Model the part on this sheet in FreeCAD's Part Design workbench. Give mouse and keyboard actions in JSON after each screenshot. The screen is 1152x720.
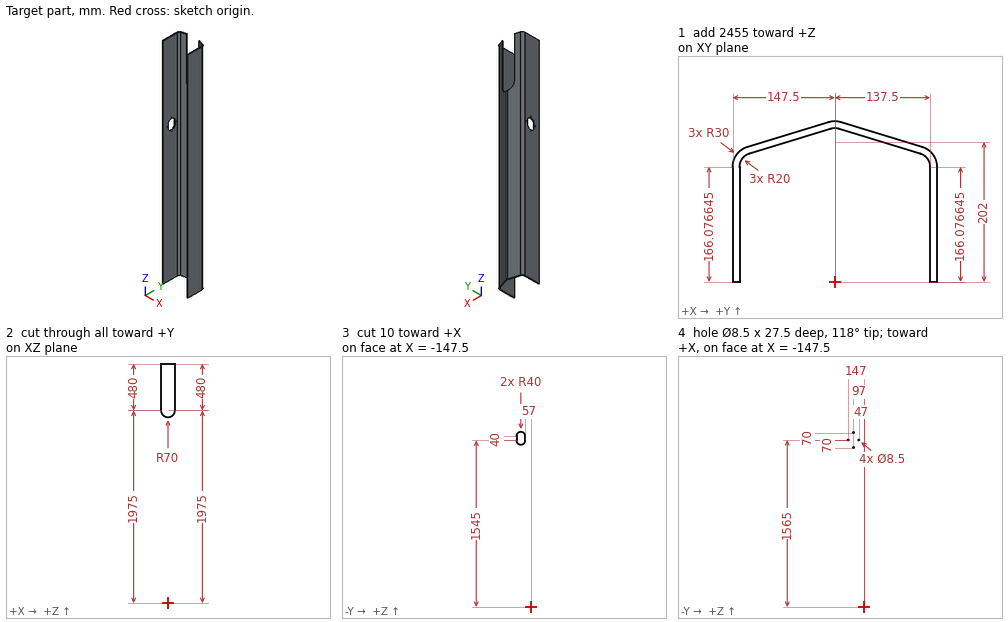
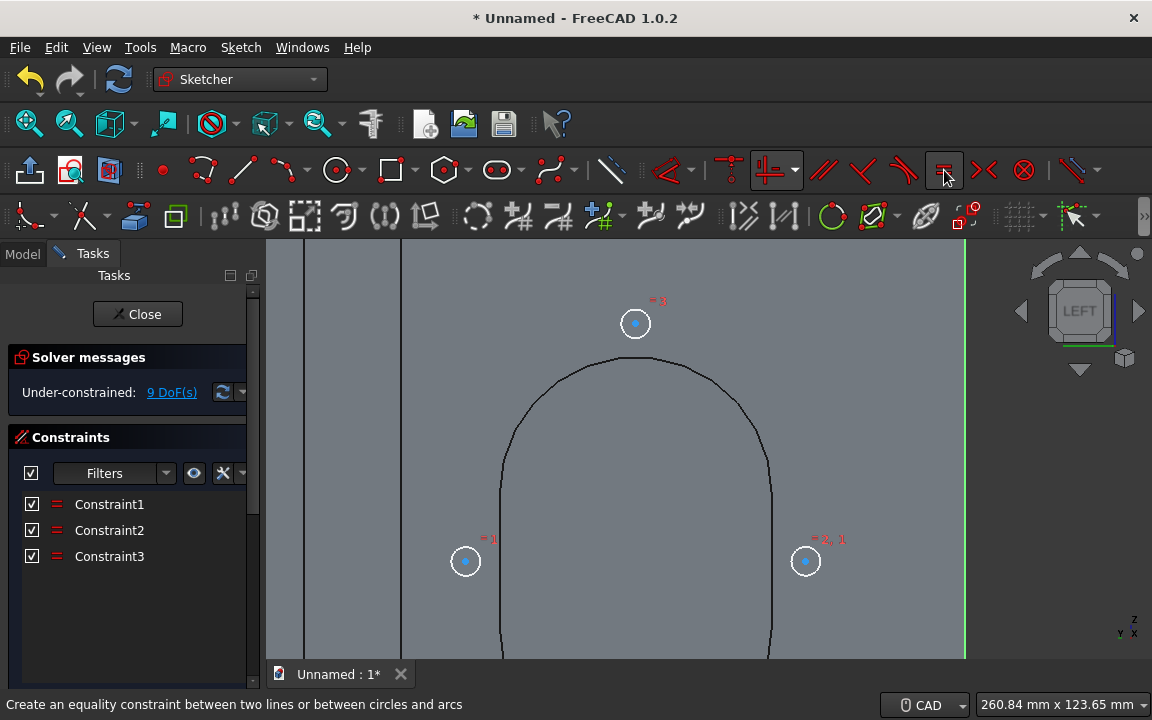
{"action": "left_click", "coordinate": [466, 561]}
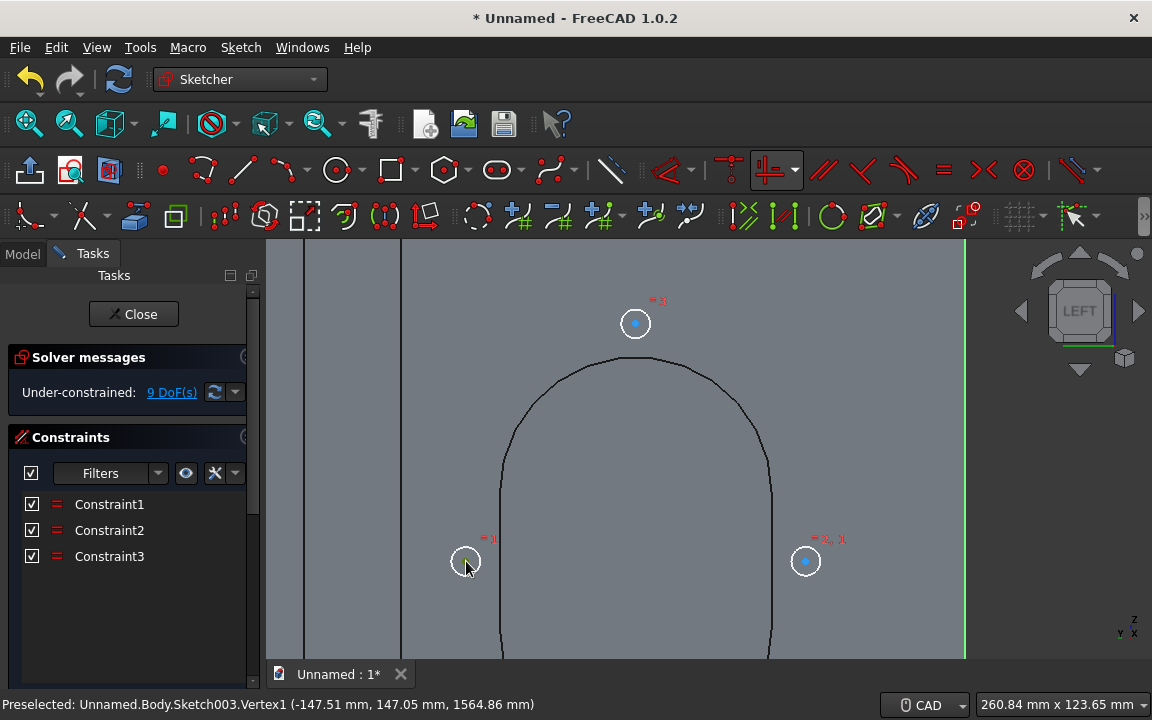
{"action": "left_click", "coordinate": [806, 561]}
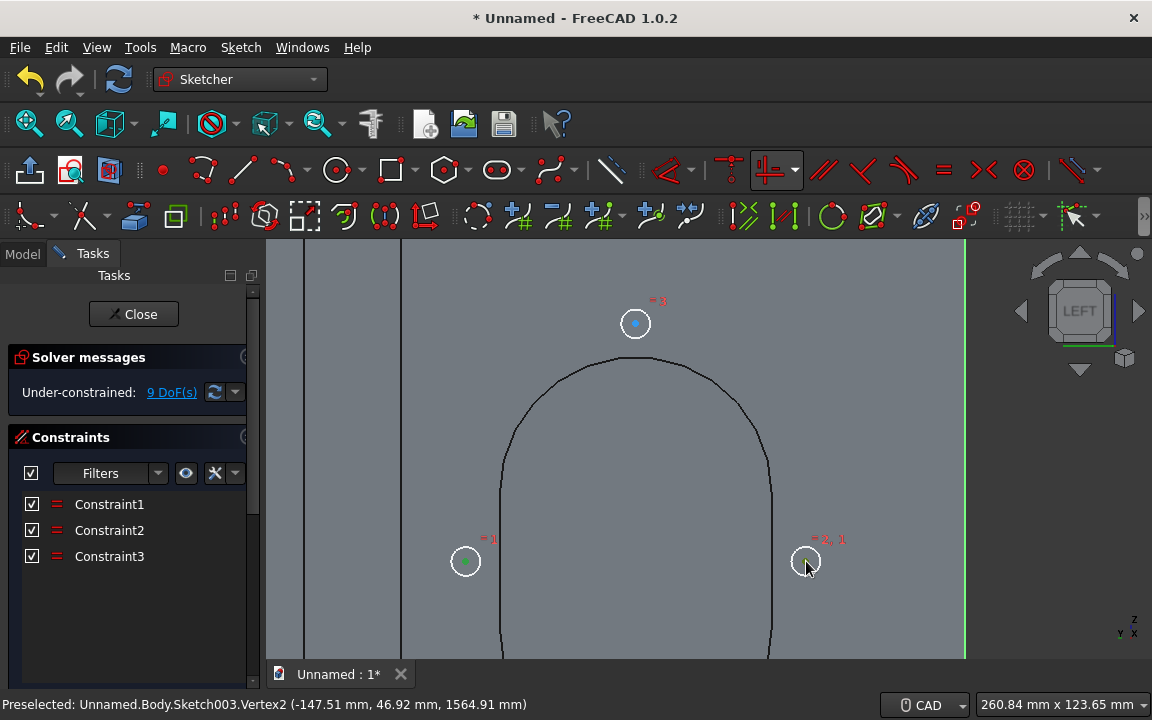
{"action": "key", "text": "h"}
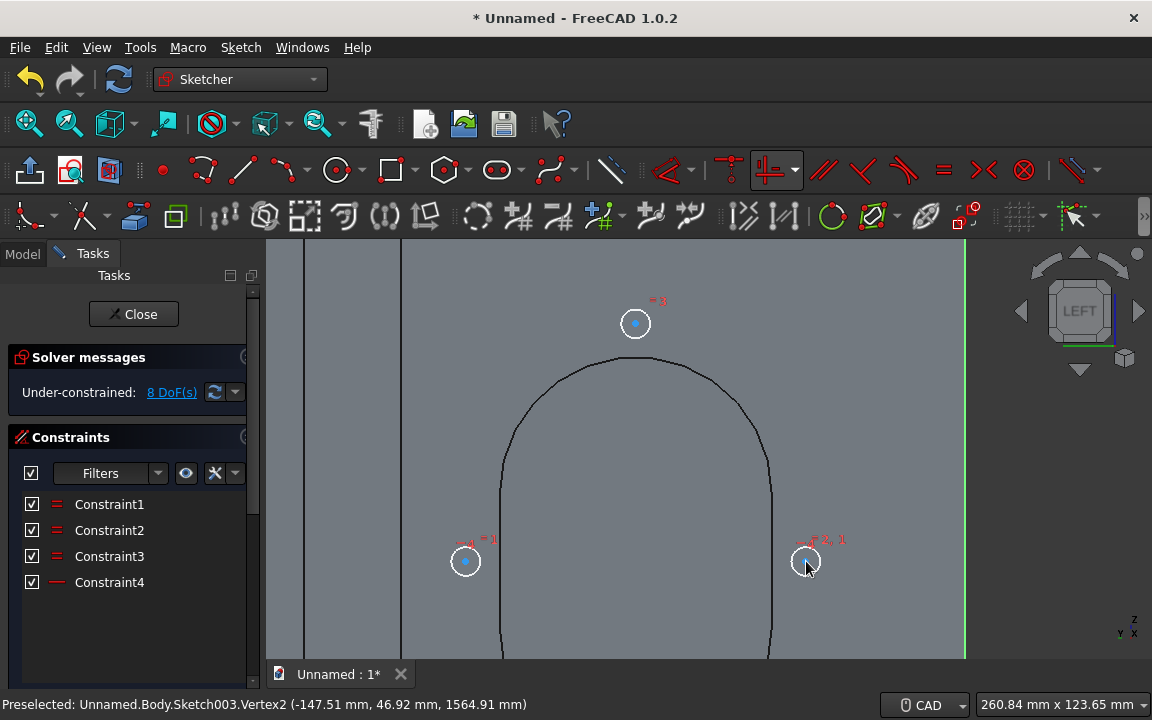
{"action": "scroll", "coordinate": [646, 313], "scroll_direction": "down", "scroll_amount": 3}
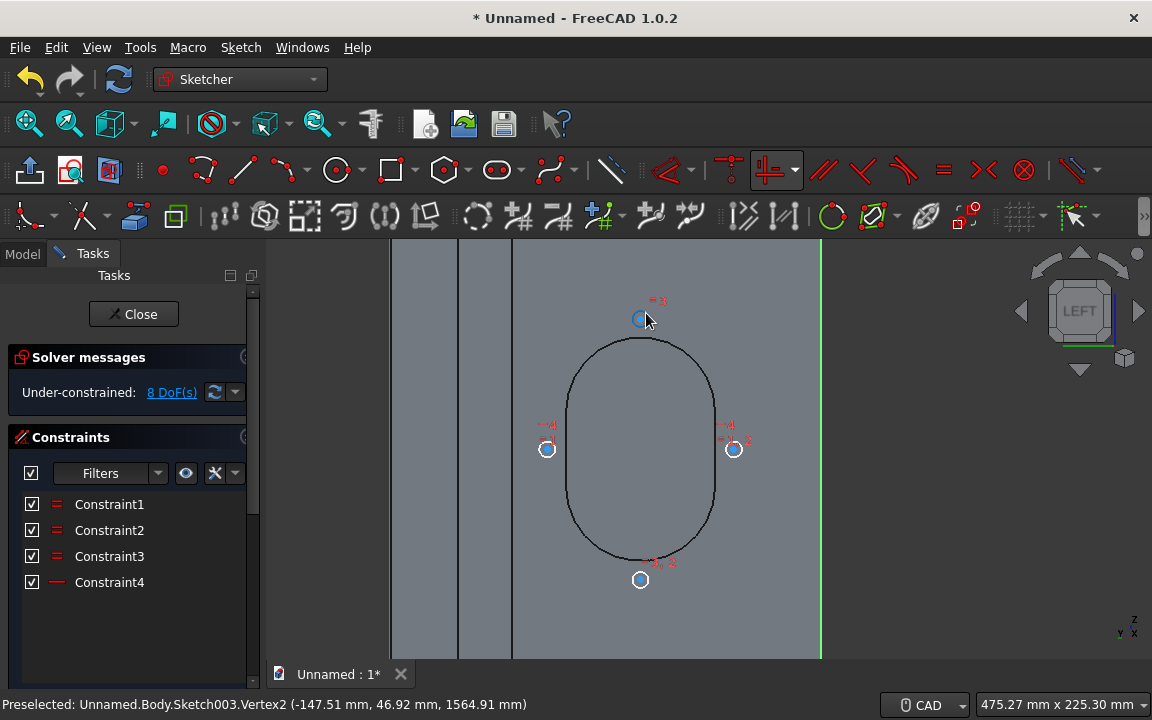
{"action": "left_click", "coordinate": [641, 580]}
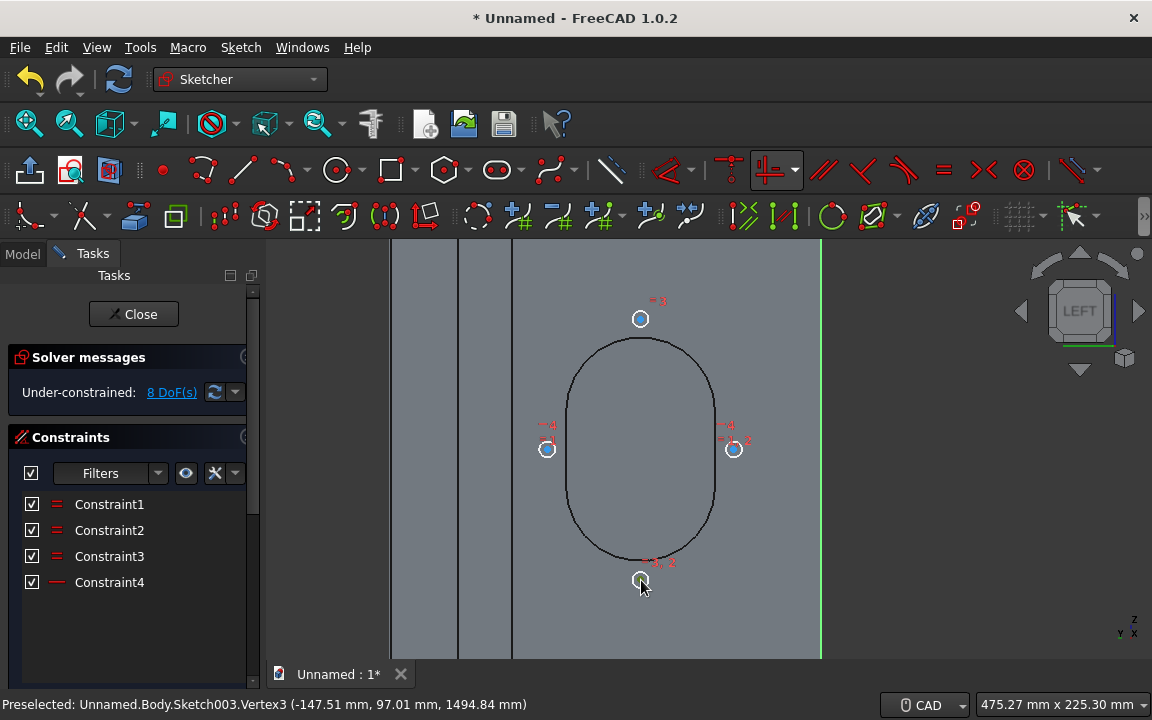
{"action": "left_click", "coordinate": [641, 319]}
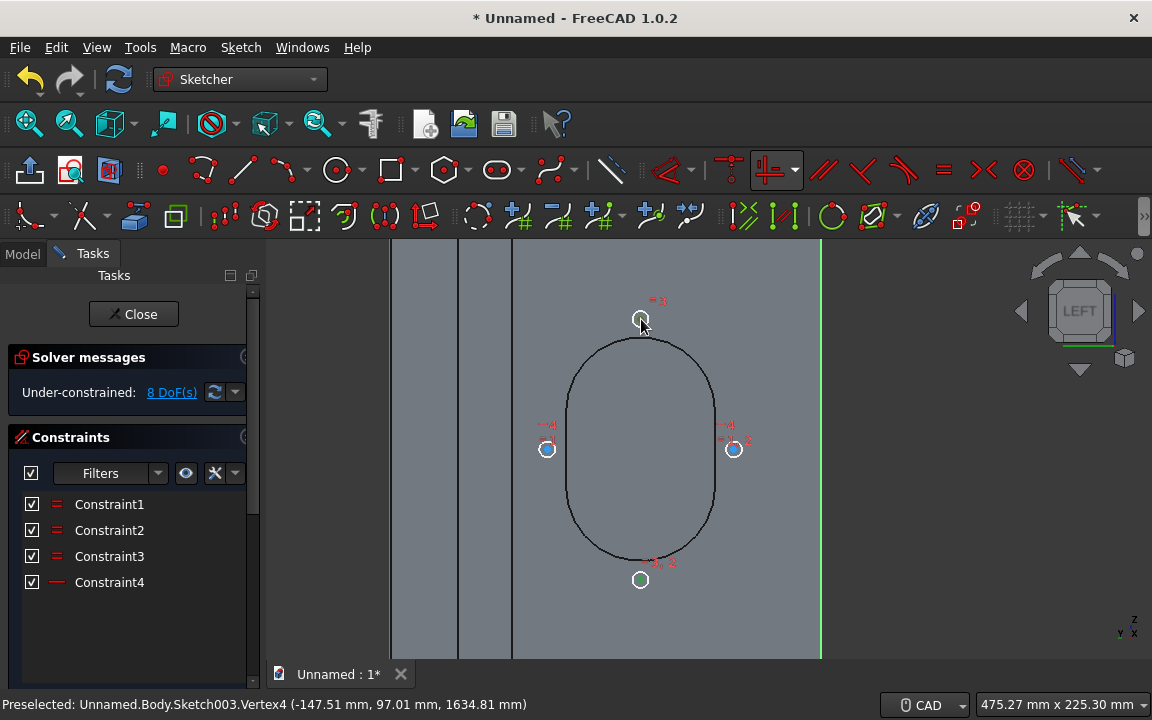
{"action": "key", "text": "v"}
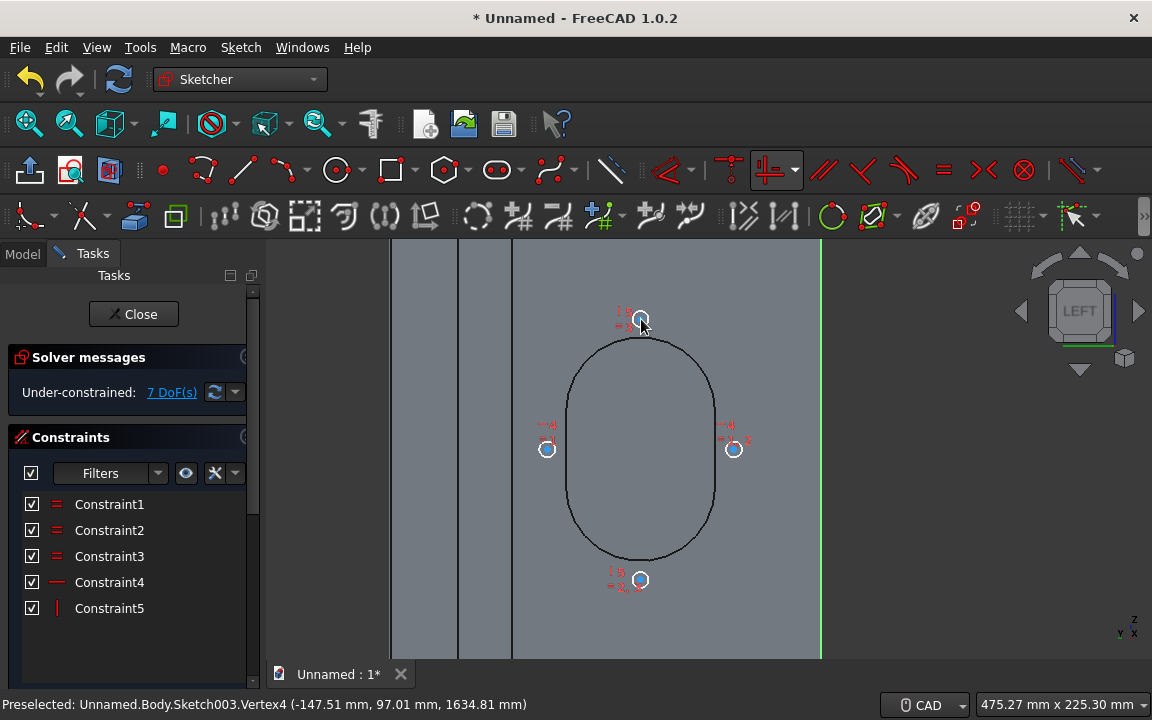
{"action": "left_click", "coordinate": [666, 170]}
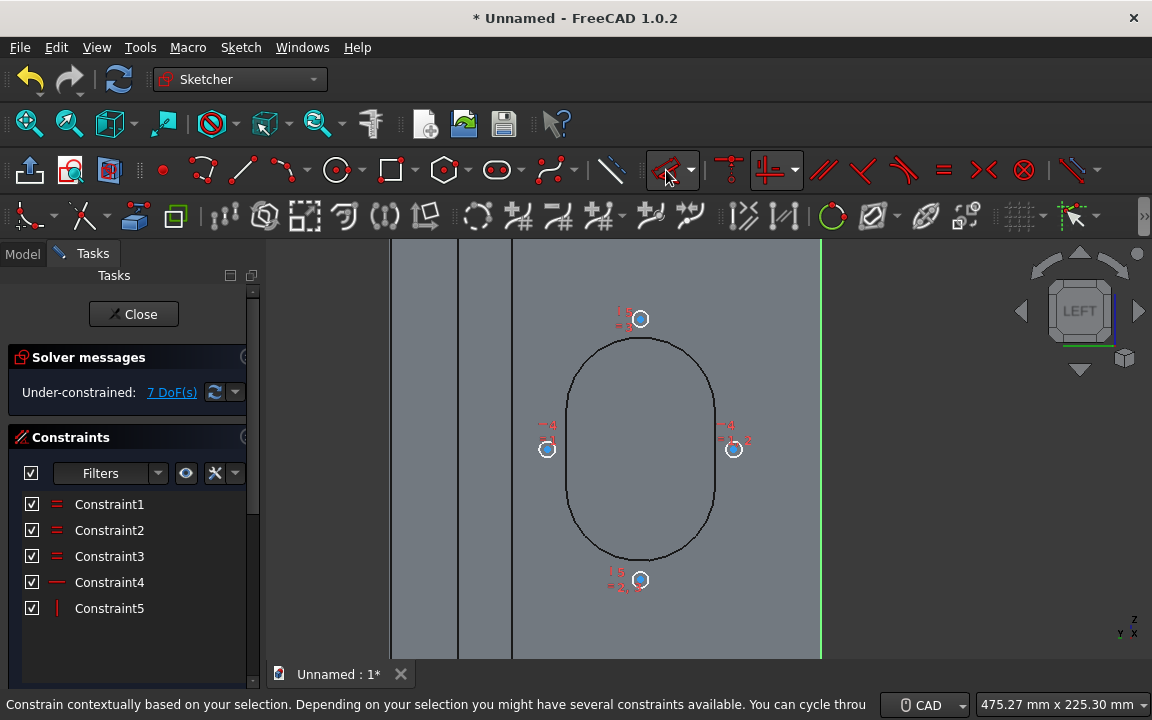
{"action": "scroll", "coordinate": [547, 442], "scroll_direction": "up", "scroll_amount": 5}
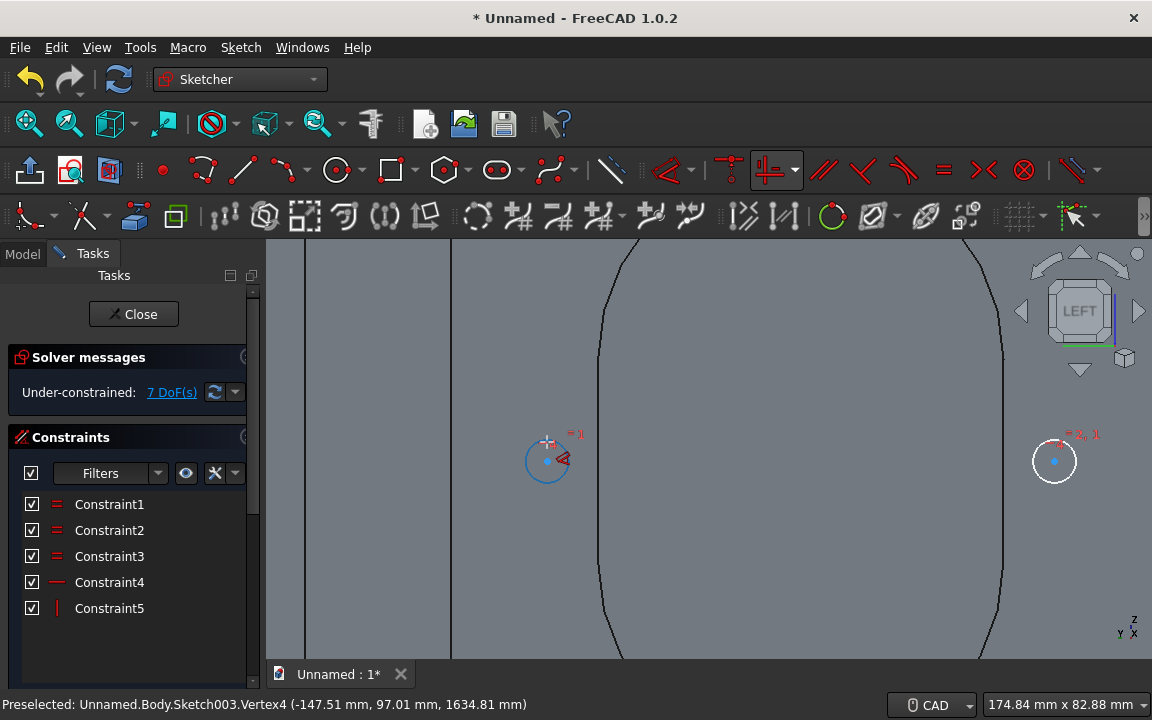
{"action": "left_click", "coordinate": [548, 440]}
{"action": "left_click", "coordinate": [549, 408]}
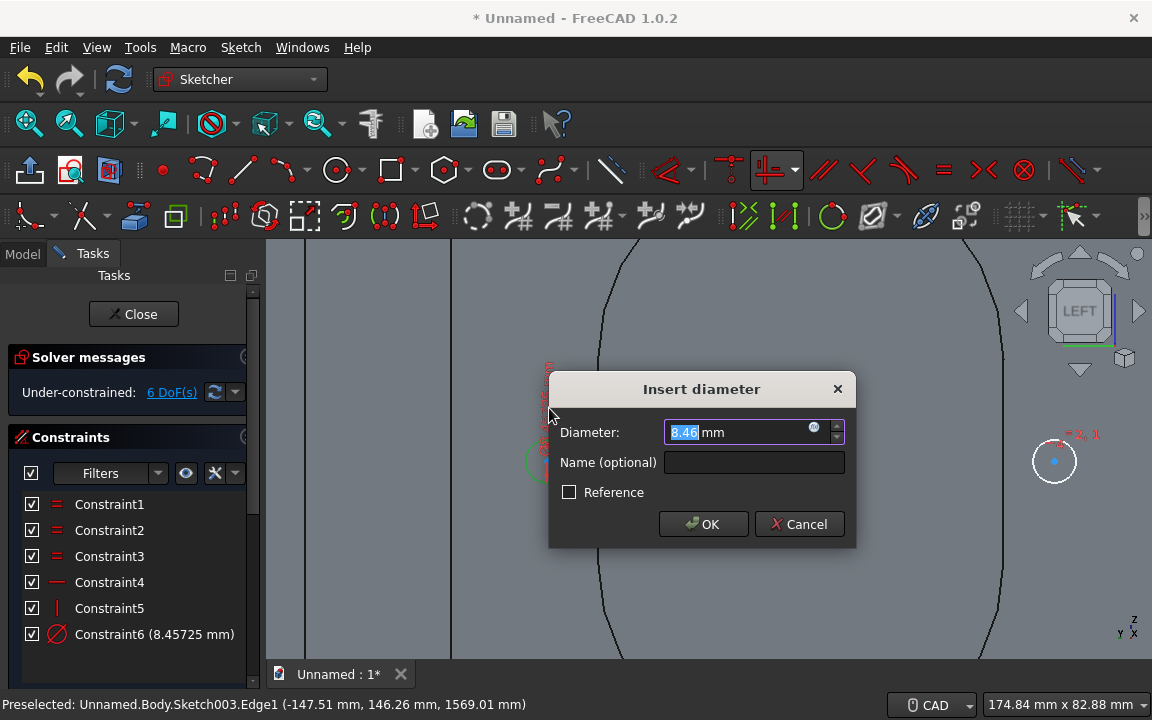
{"action": "type", "text": "8.5"}
{"action": "key", "text": "Return"}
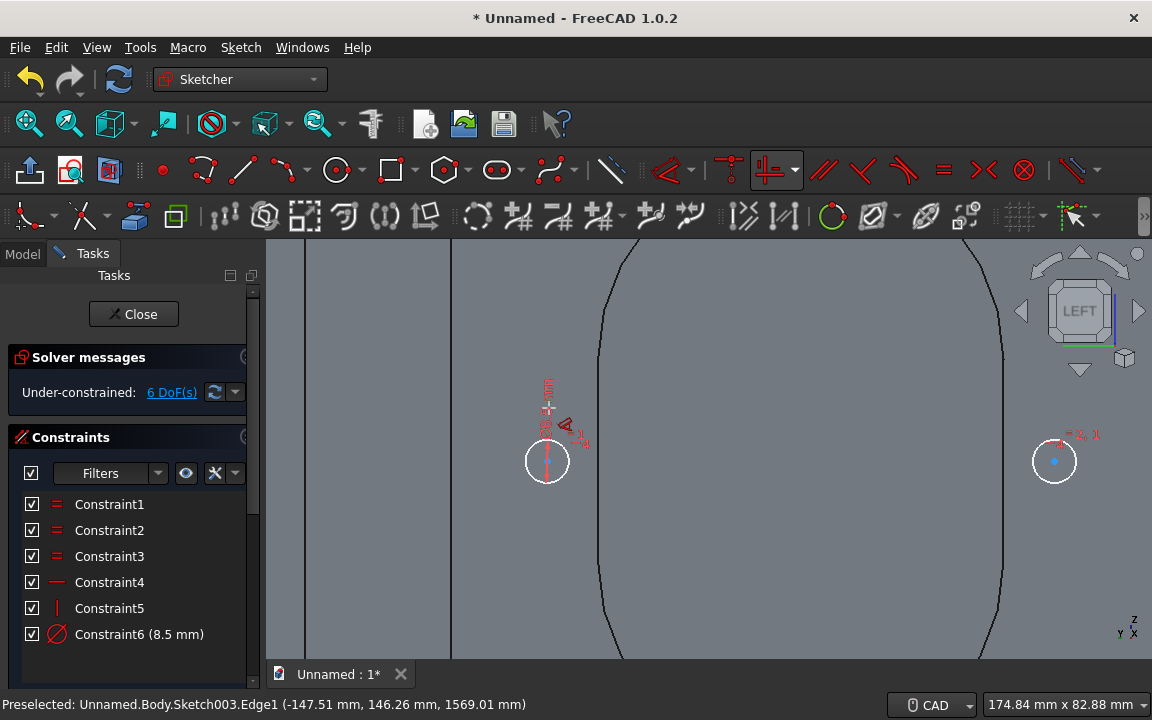
{"action": "scroll", "coordinate": [547, 442], "scroll_direction": "down", "scroll_amount": 5}